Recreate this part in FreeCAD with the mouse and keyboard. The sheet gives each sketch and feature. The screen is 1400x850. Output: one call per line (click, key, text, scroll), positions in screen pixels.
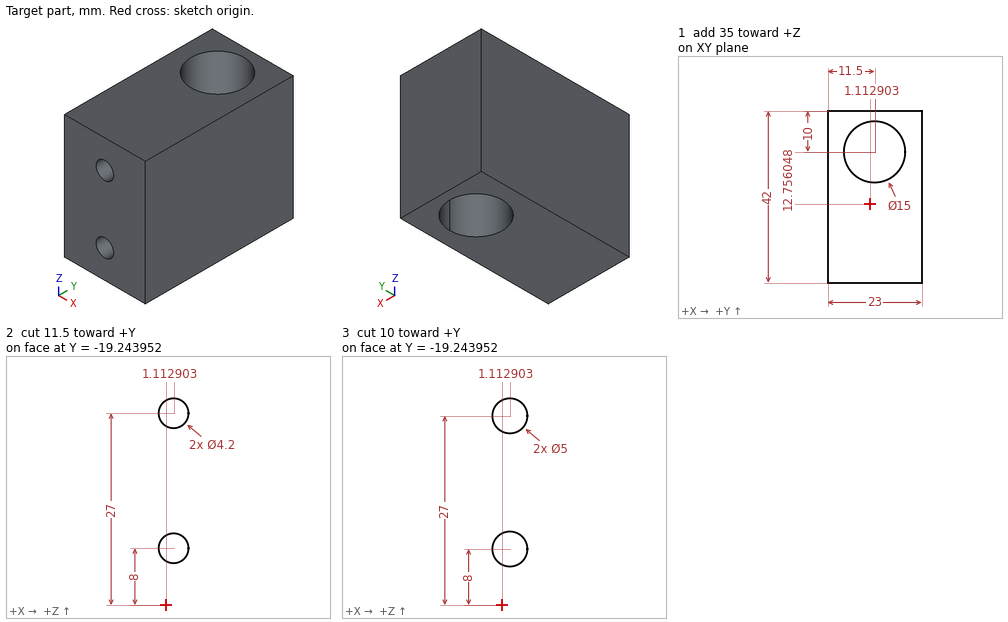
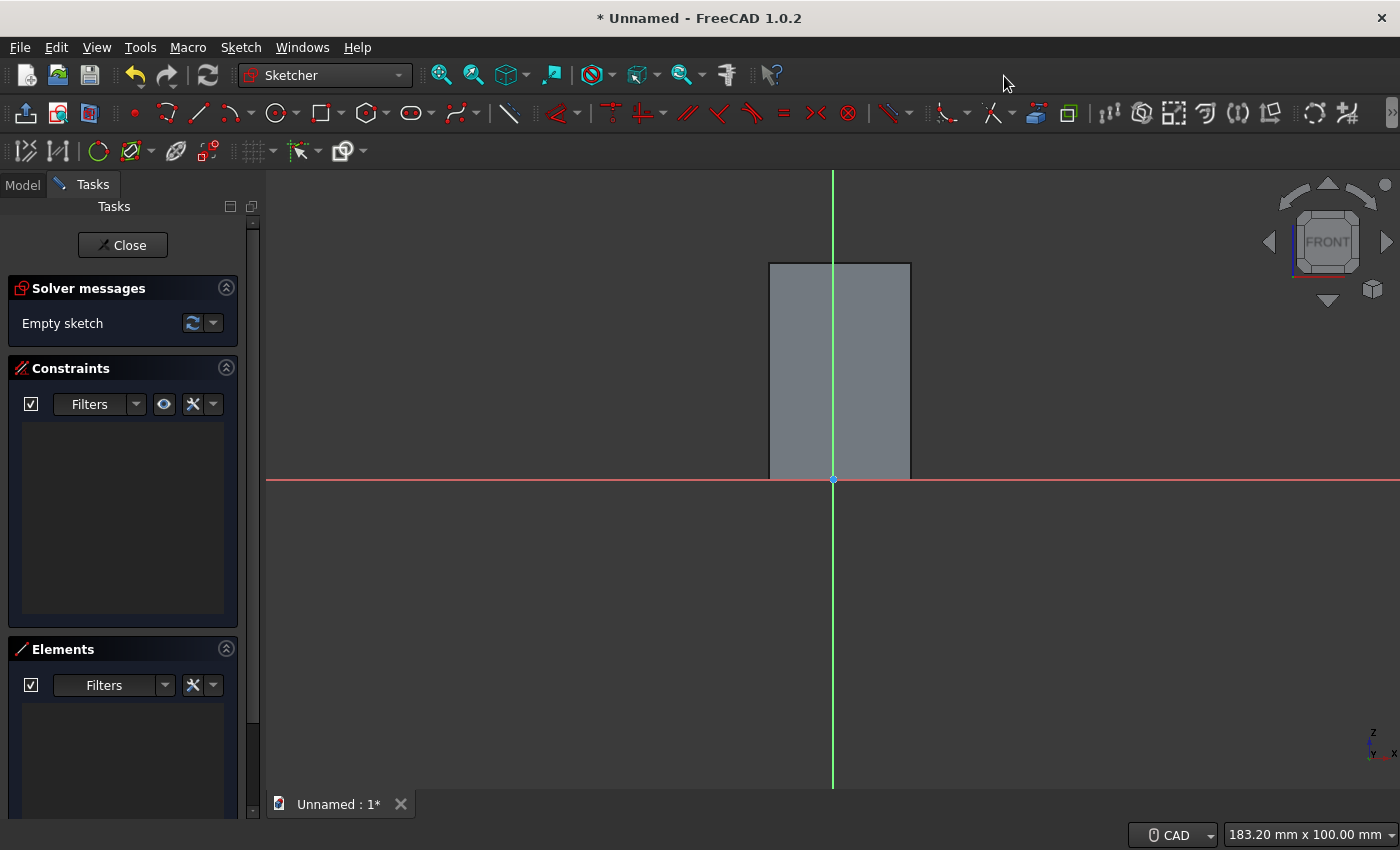
scroll(901, 316, up, 4)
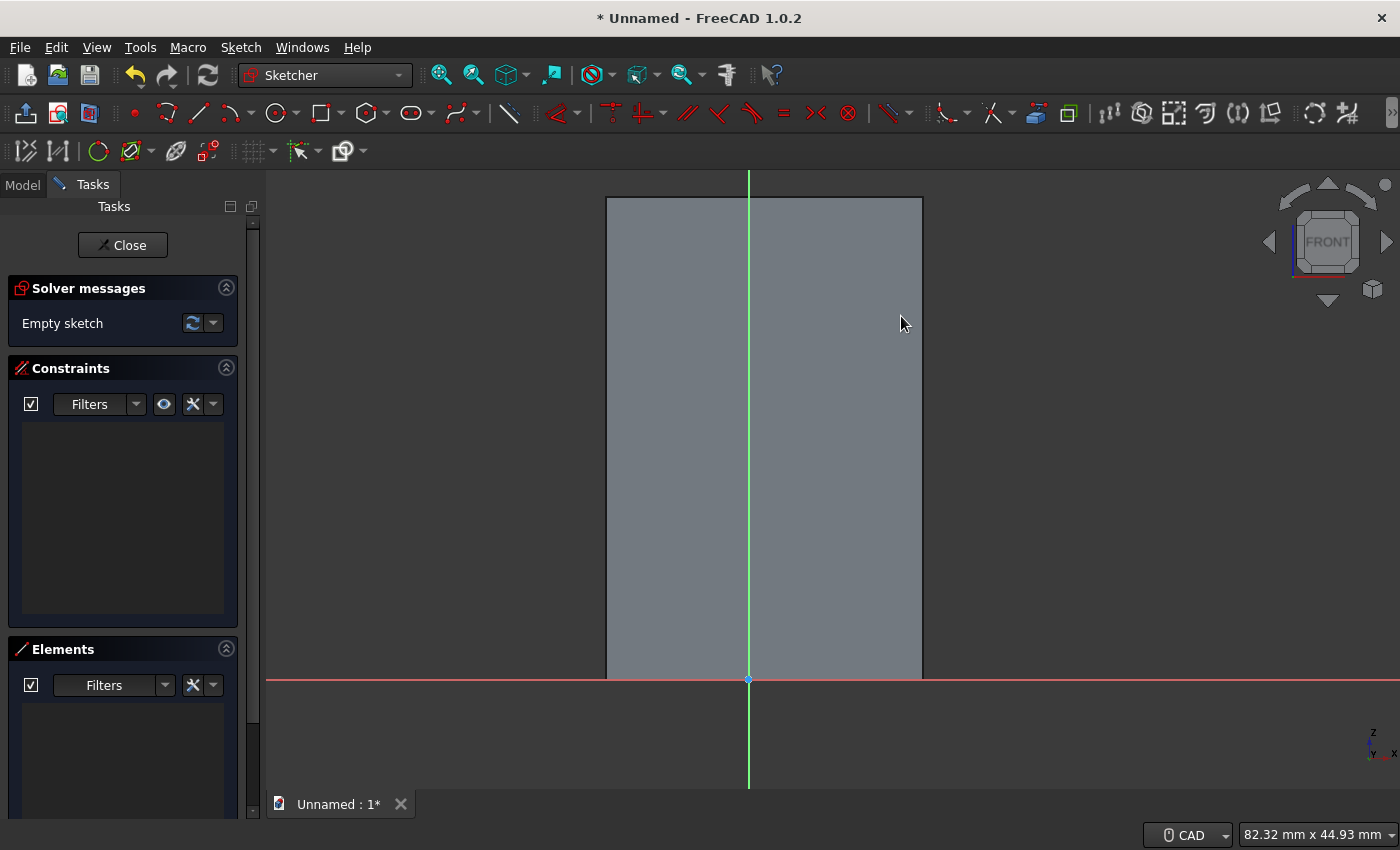
click(276, 114)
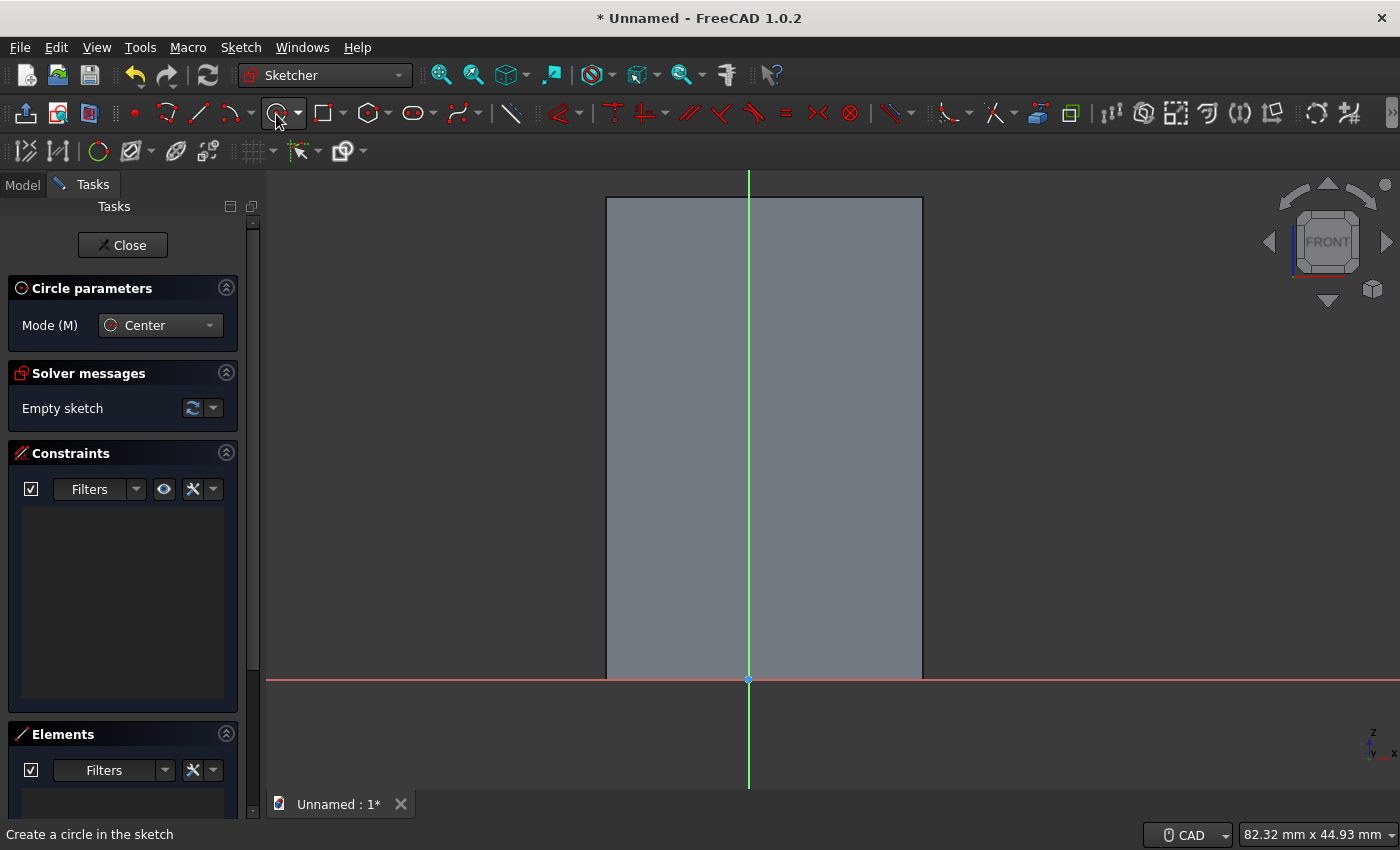
click(764, 308)
click(785, 287)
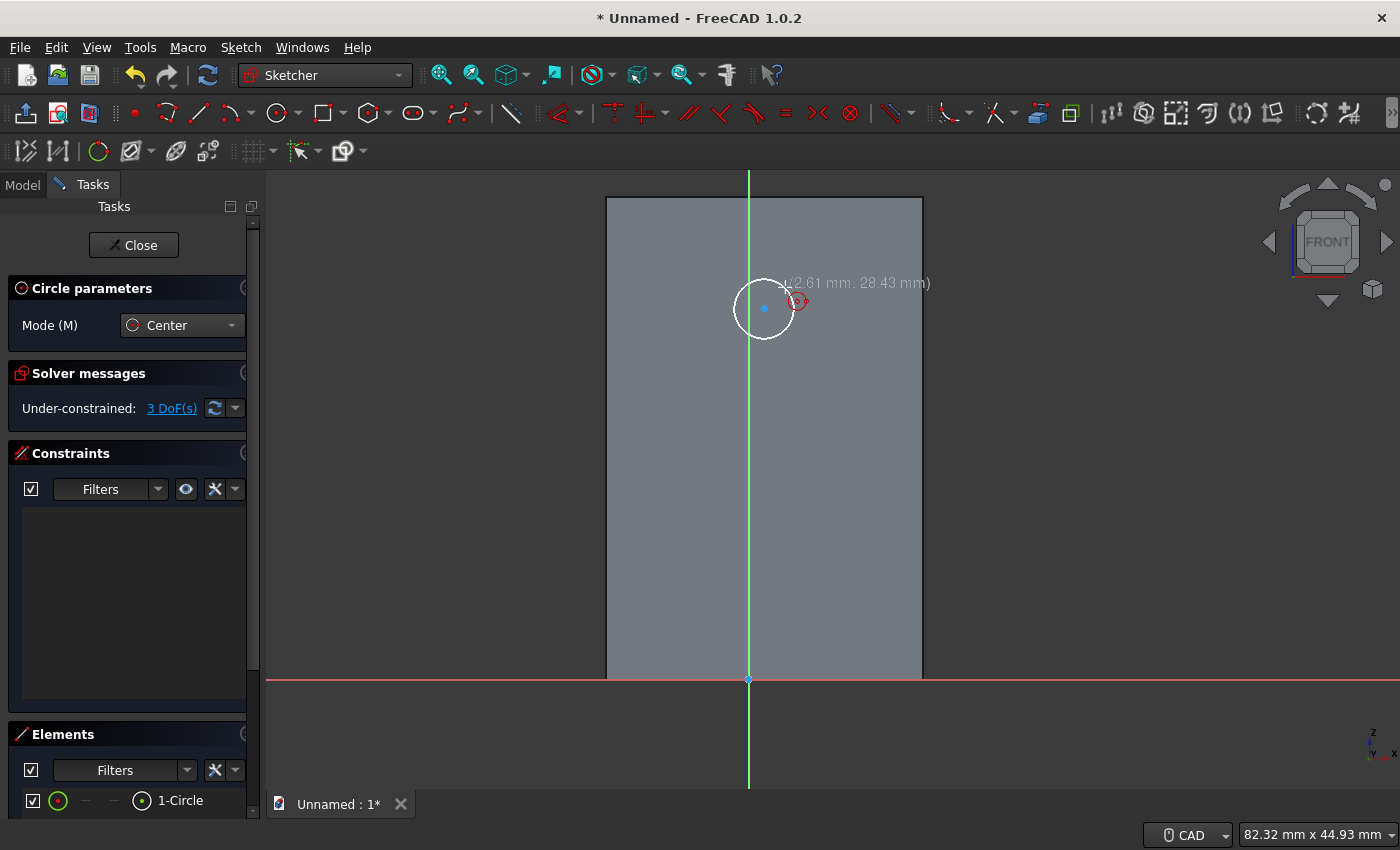
click(764, 569)
click(785, 549)
key(Escape)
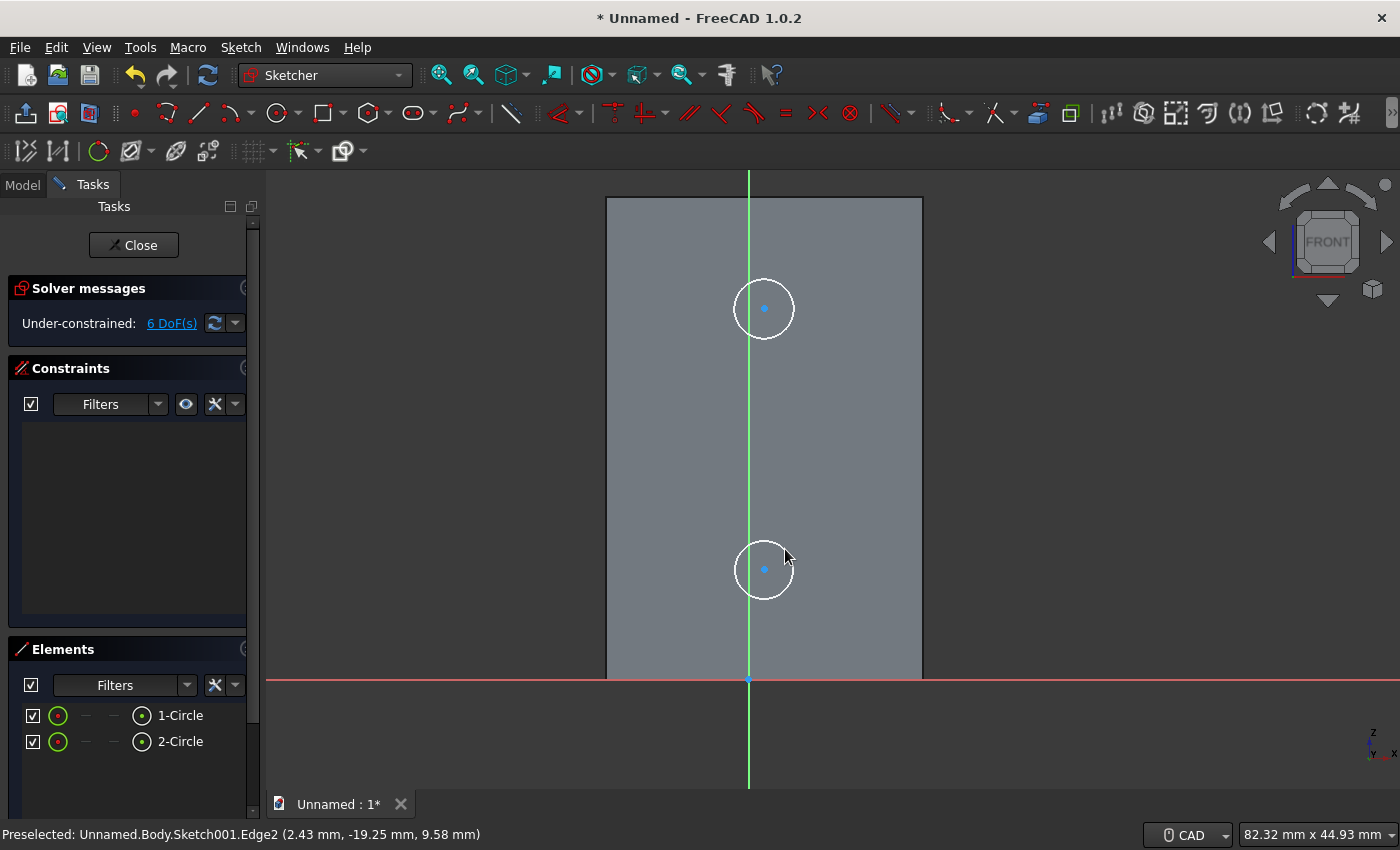
click(785, 288)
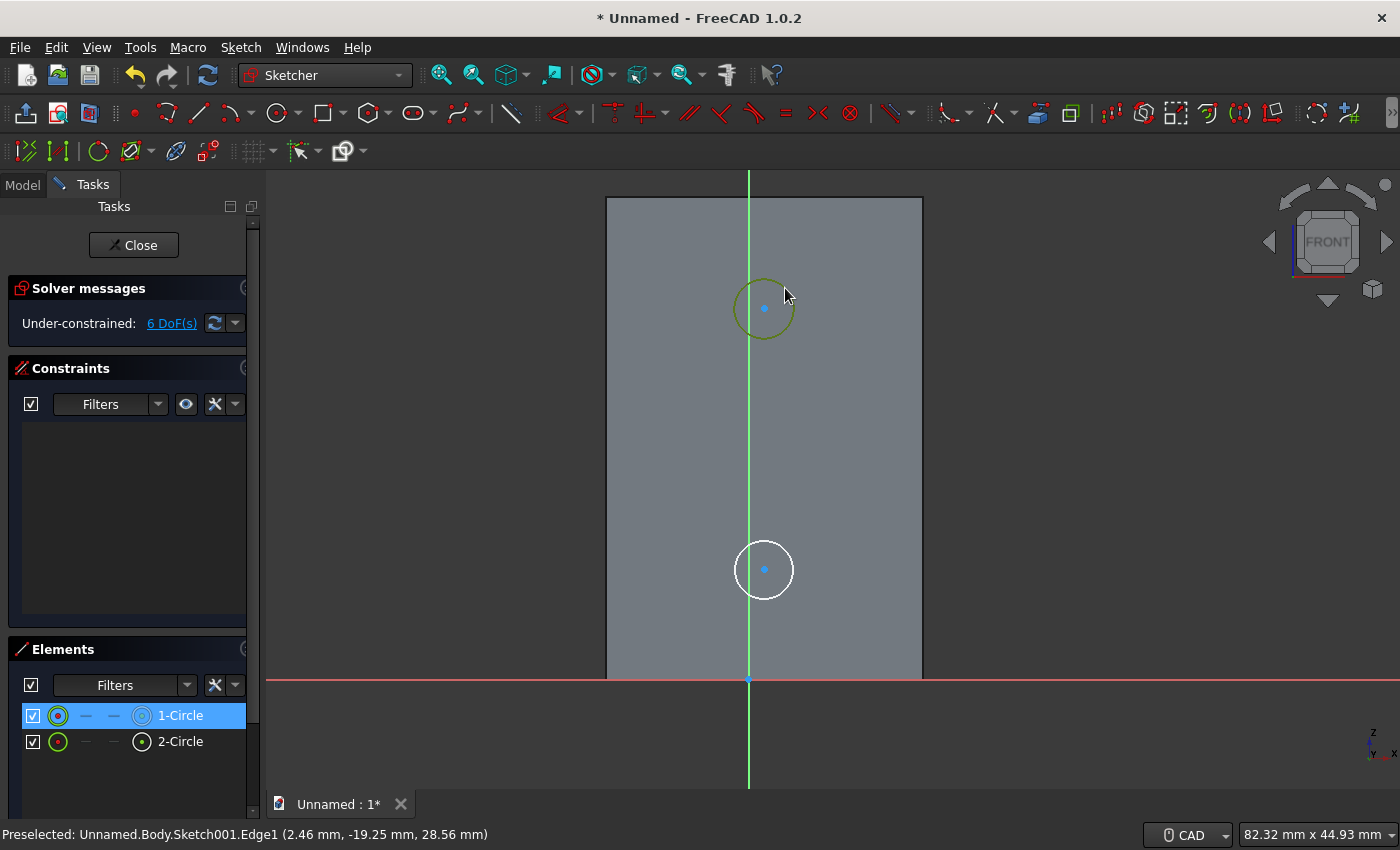
click(784, 549)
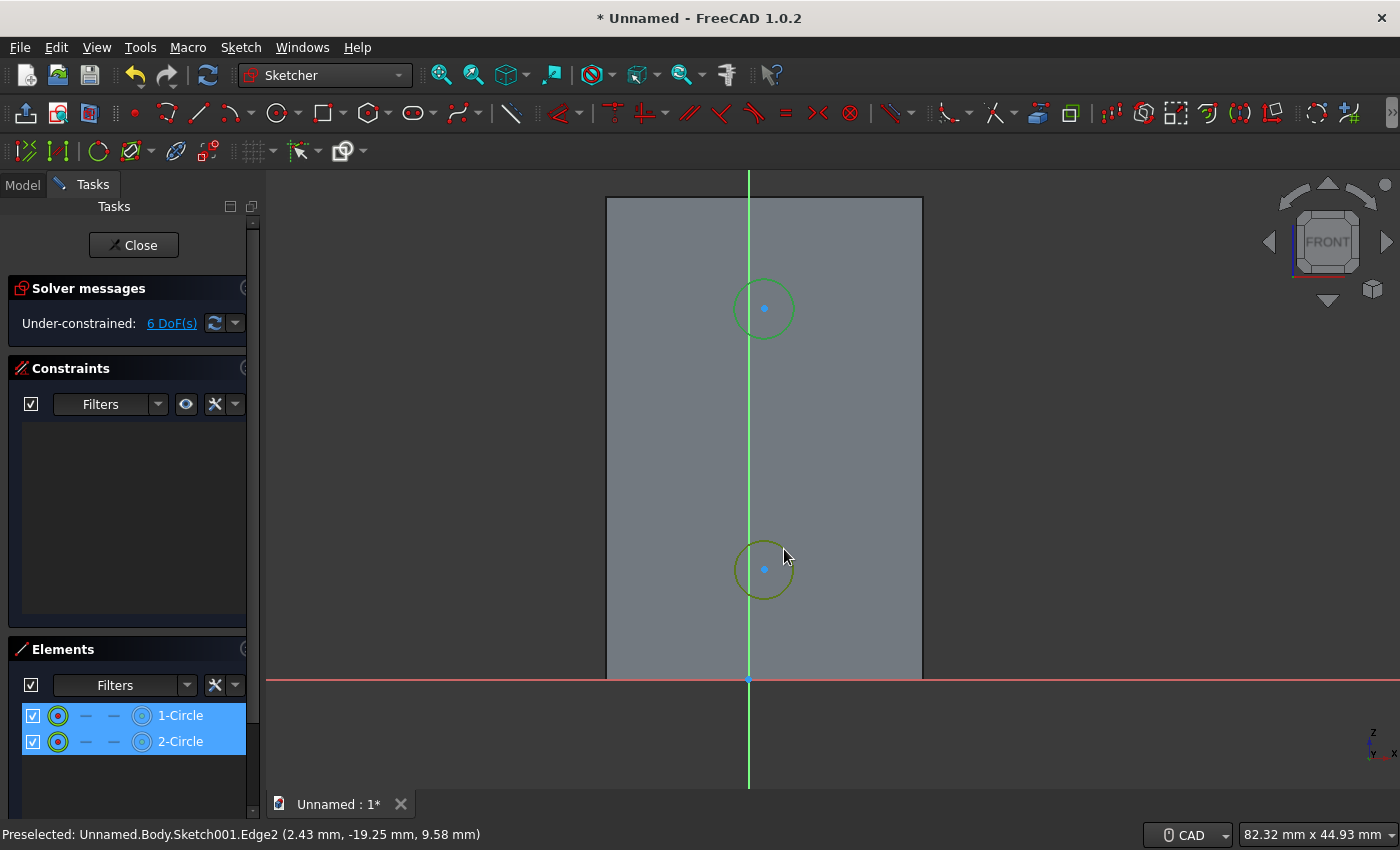
click(786, 114)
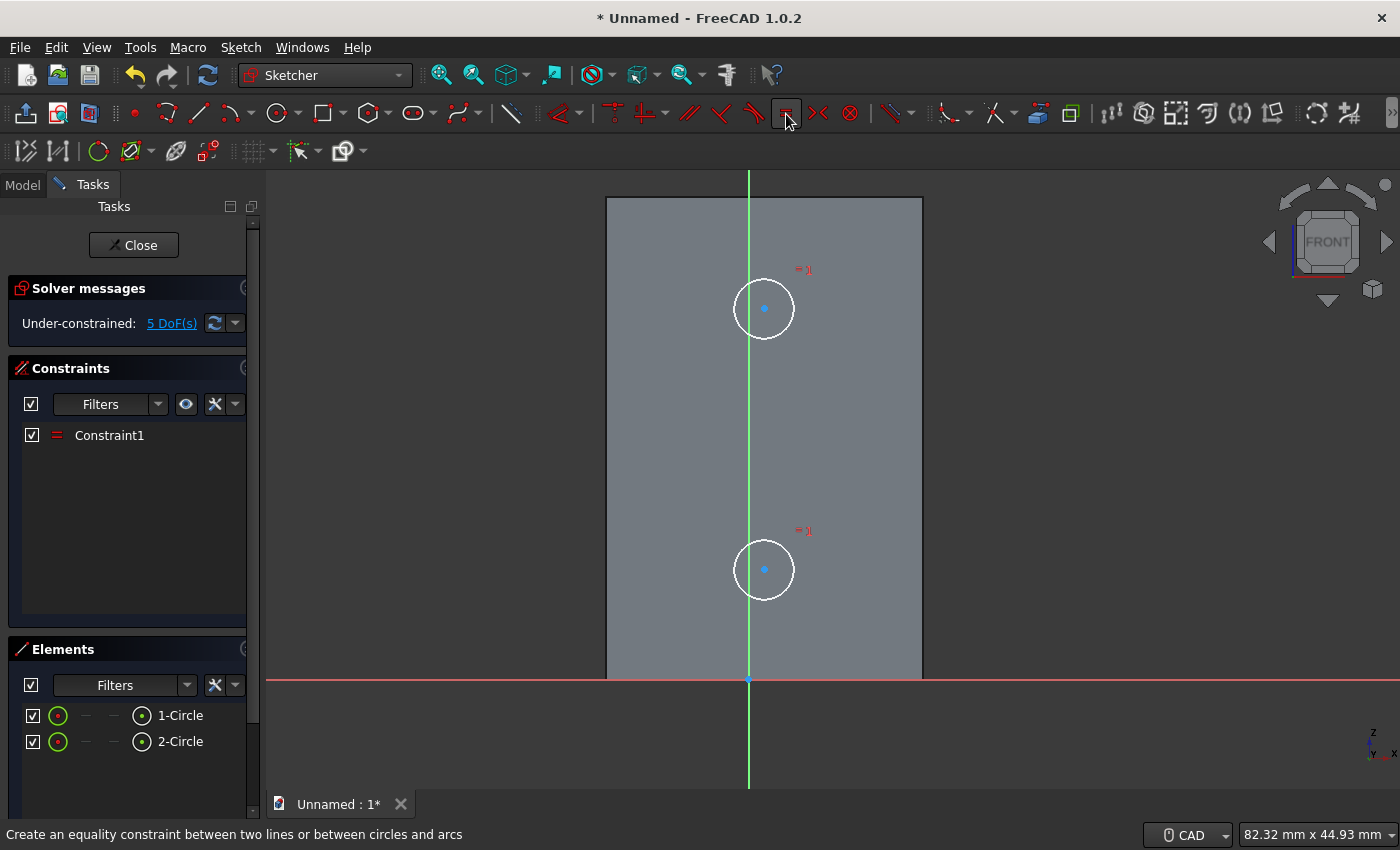
click(764, 309)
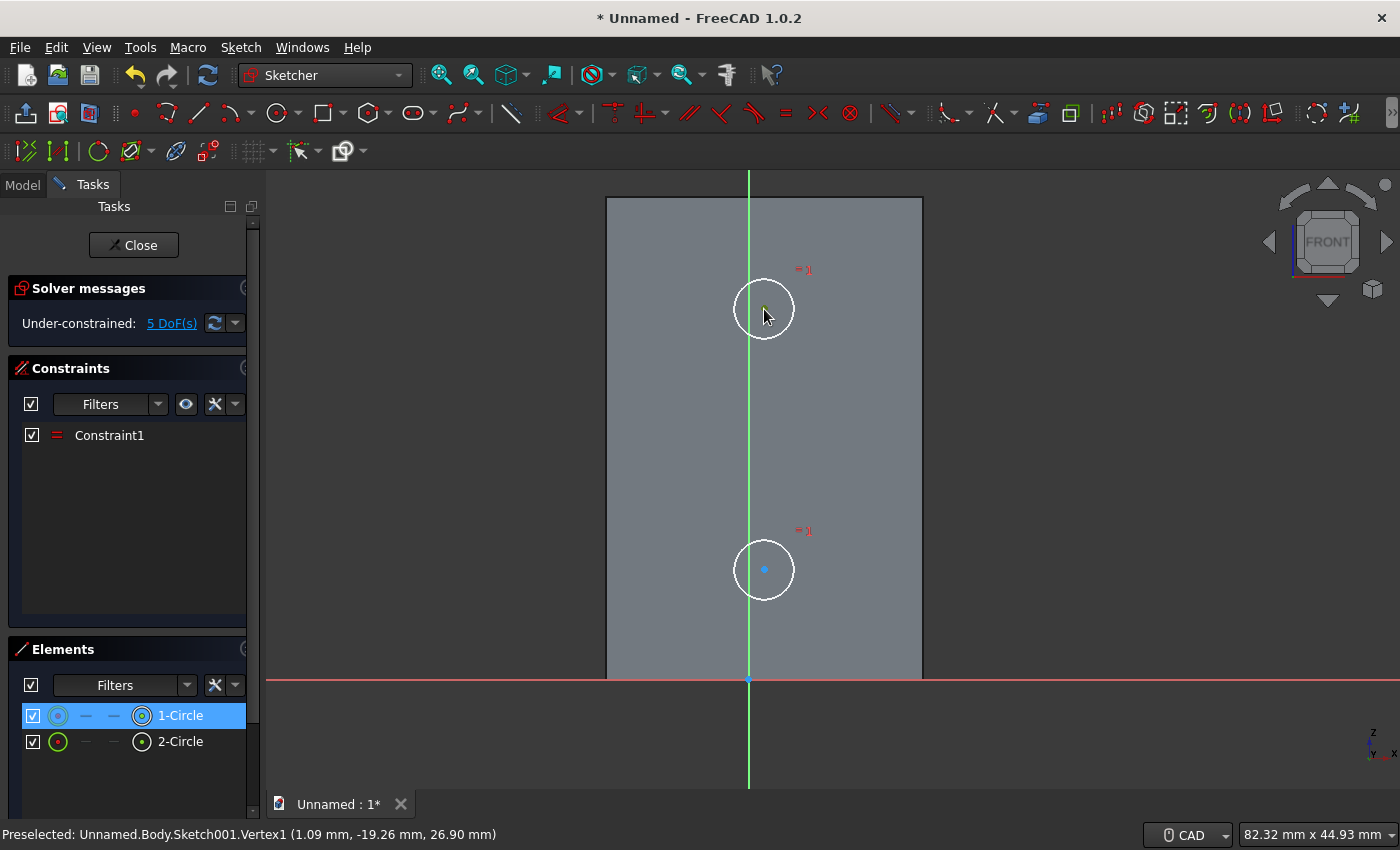
click(764, 570)